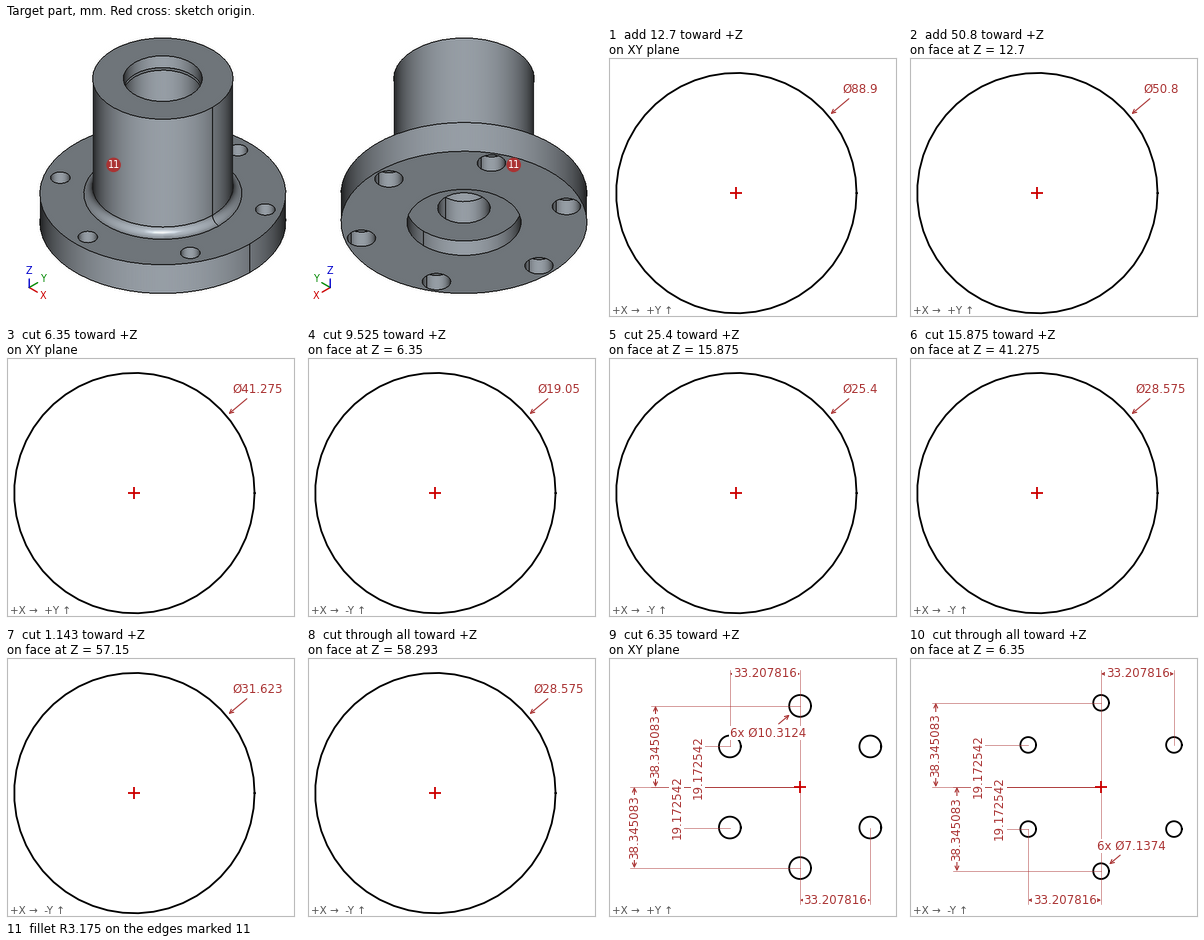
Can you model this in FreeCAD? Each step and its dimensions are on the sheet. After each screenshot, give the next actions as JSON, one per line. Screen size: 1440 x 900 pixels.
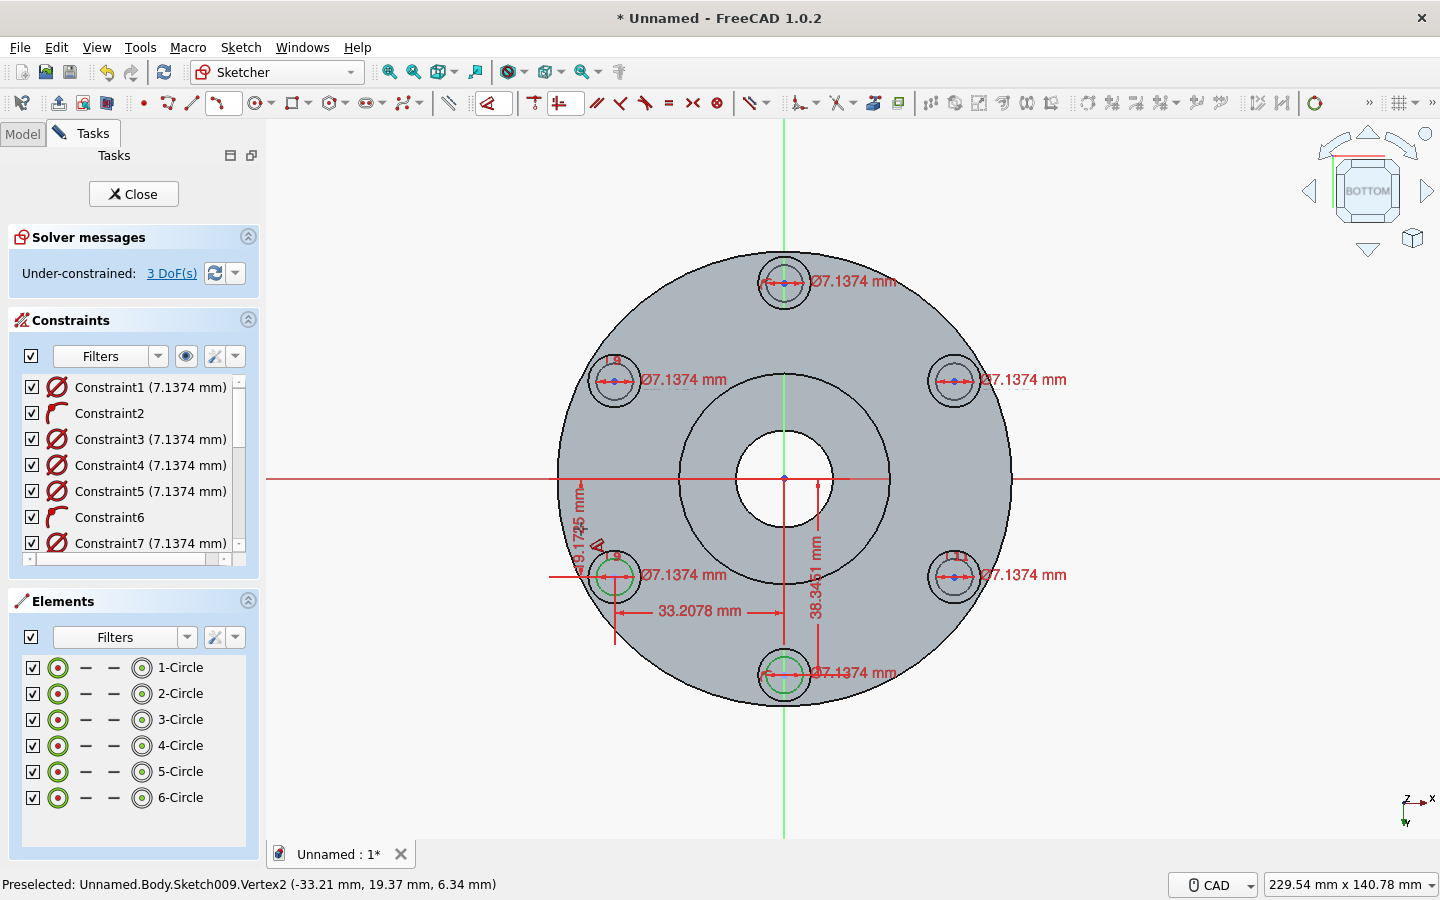
{"action": "left_click", "coordinate": [615, 382]}
{"action": "left_click", "coordinate": [581, 430]}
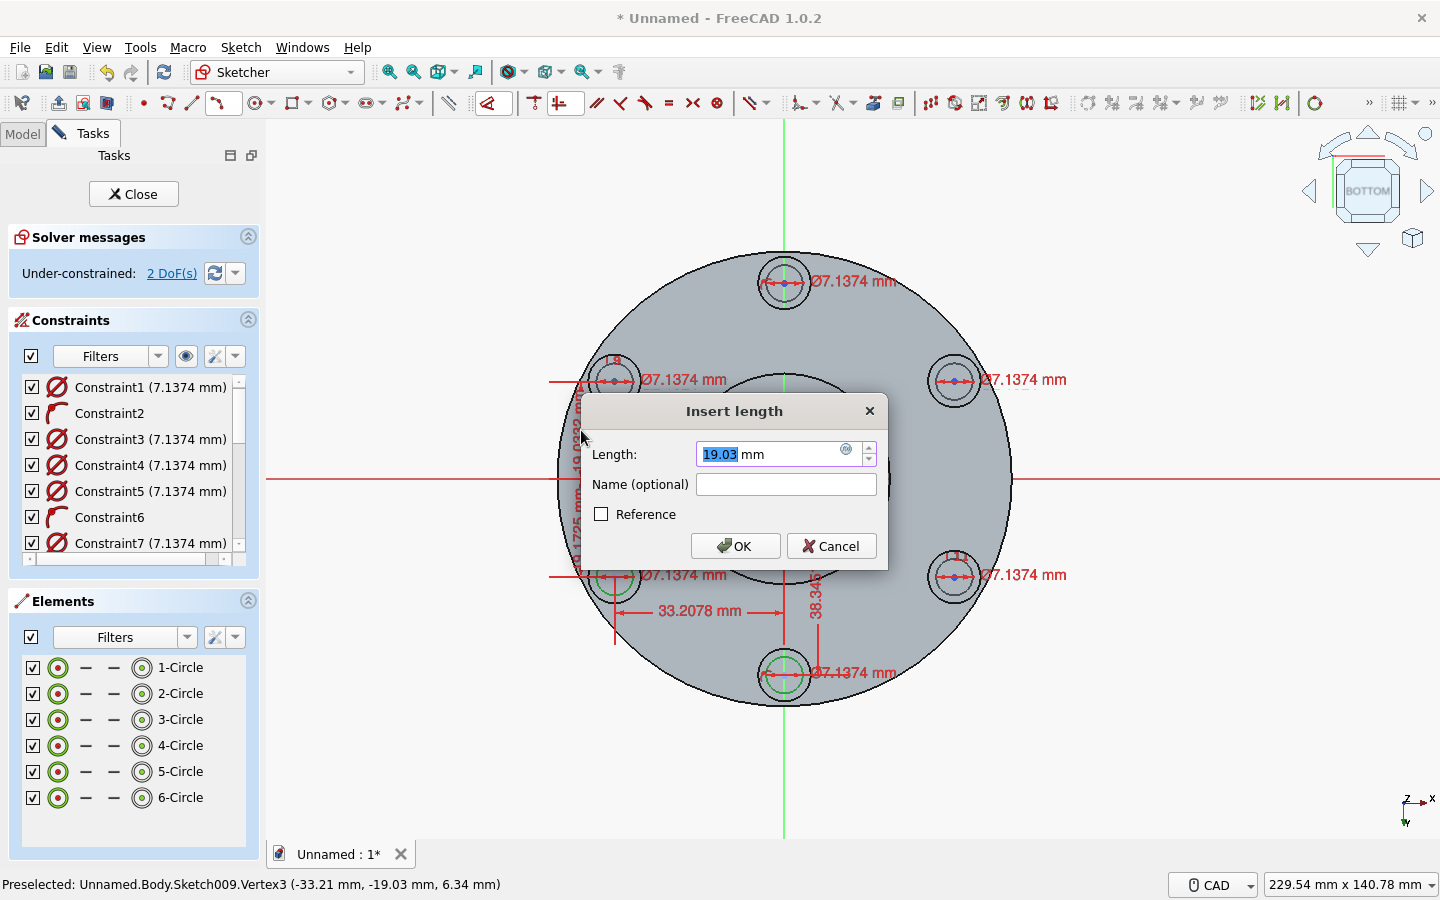
{"action": "type", "text": "19.172542"}
{"action": "key", "text": "Return"}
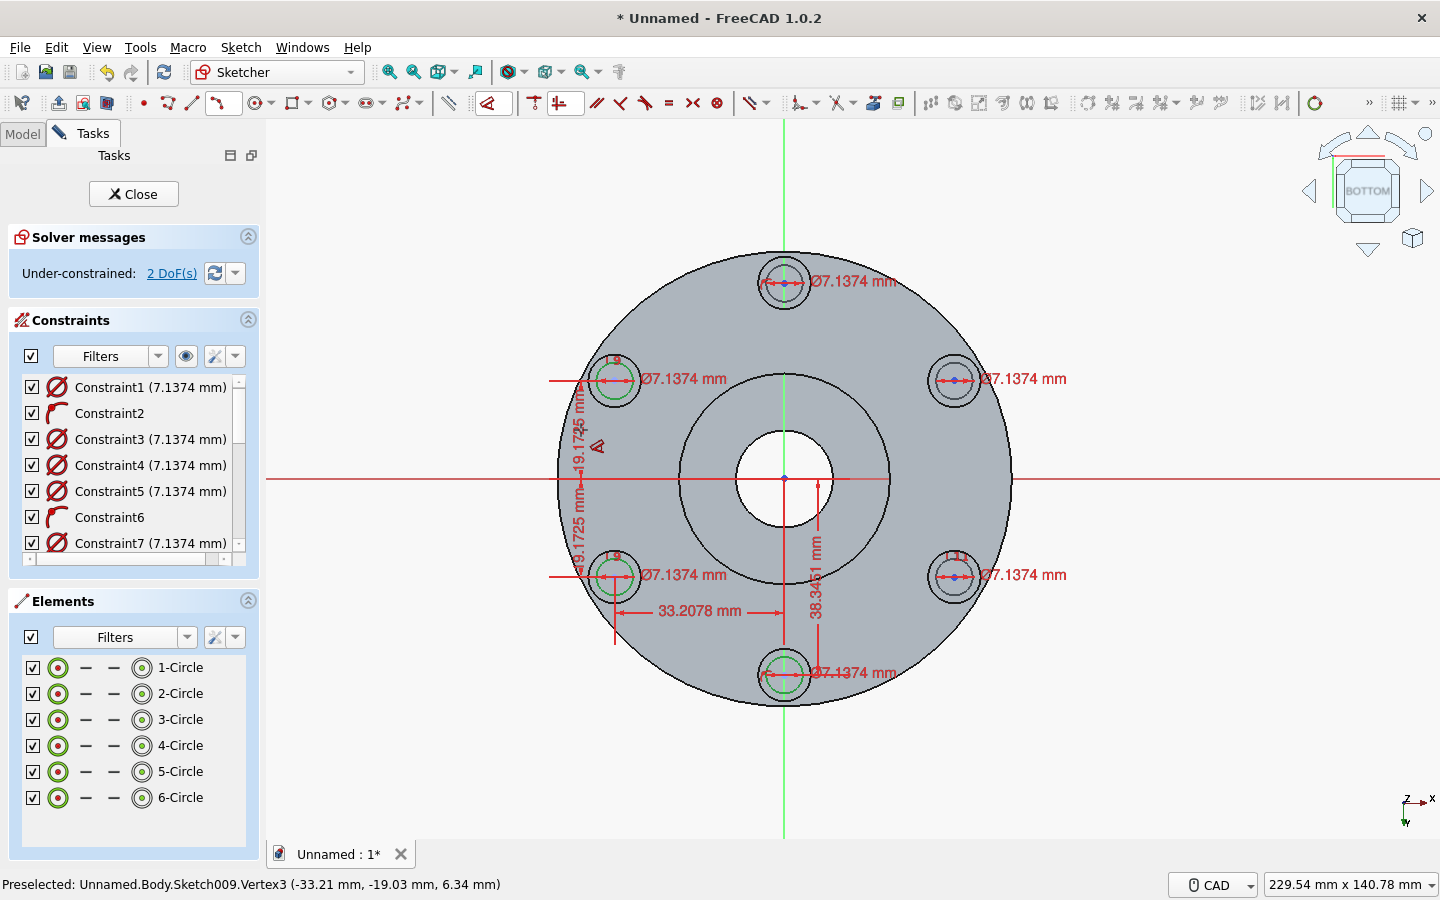
{"action": "left_click", "coordinate": [784, 283]}
{"action": "left_click", "coordinate": [818, 381]}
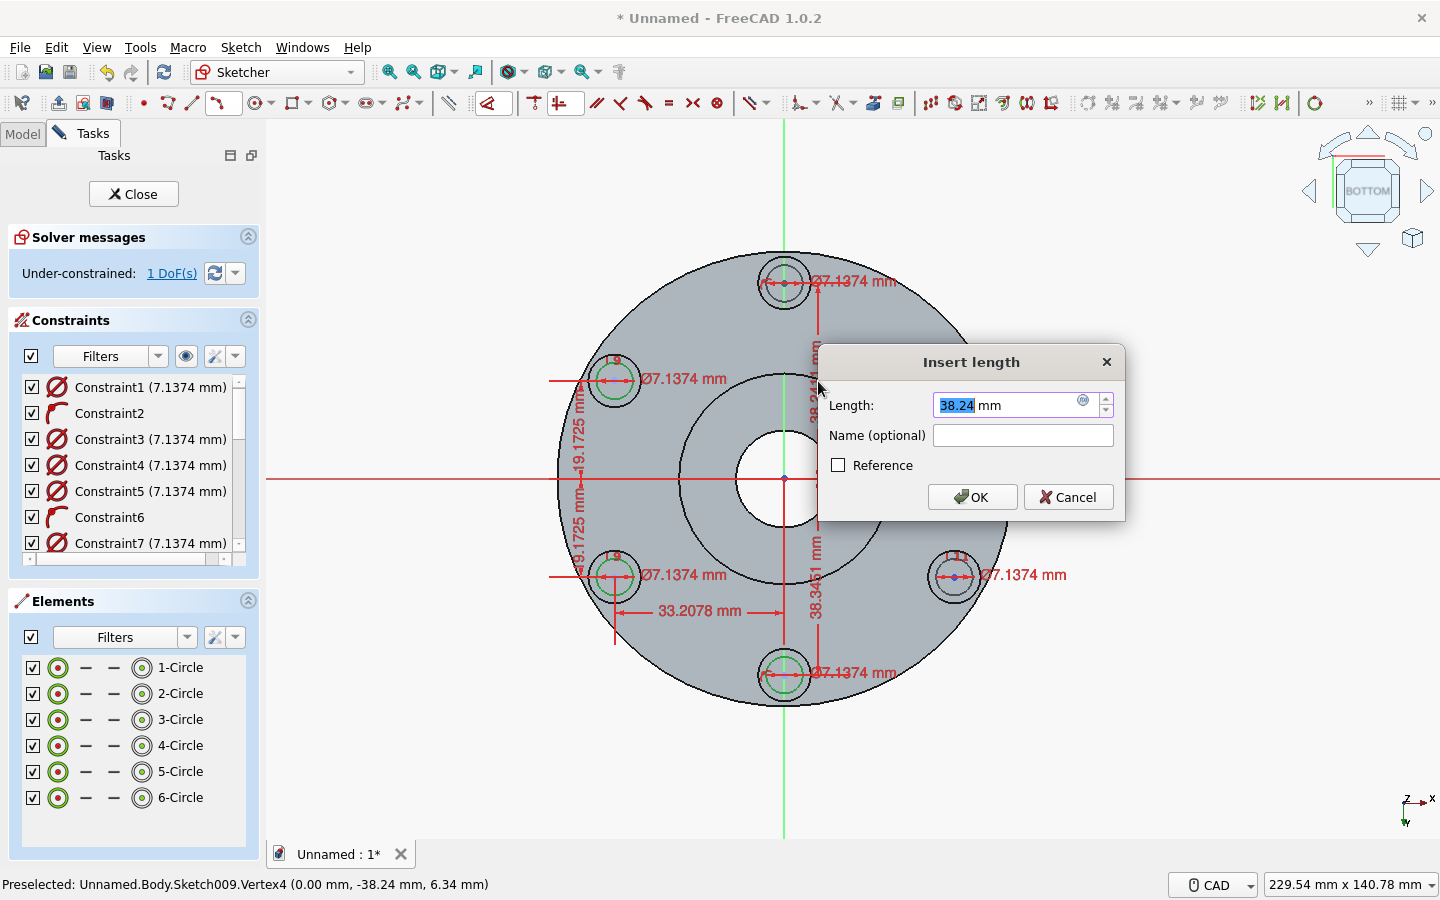
{"action": "type", "text": "38.345083"}
{"action": "key", "text": "Return"}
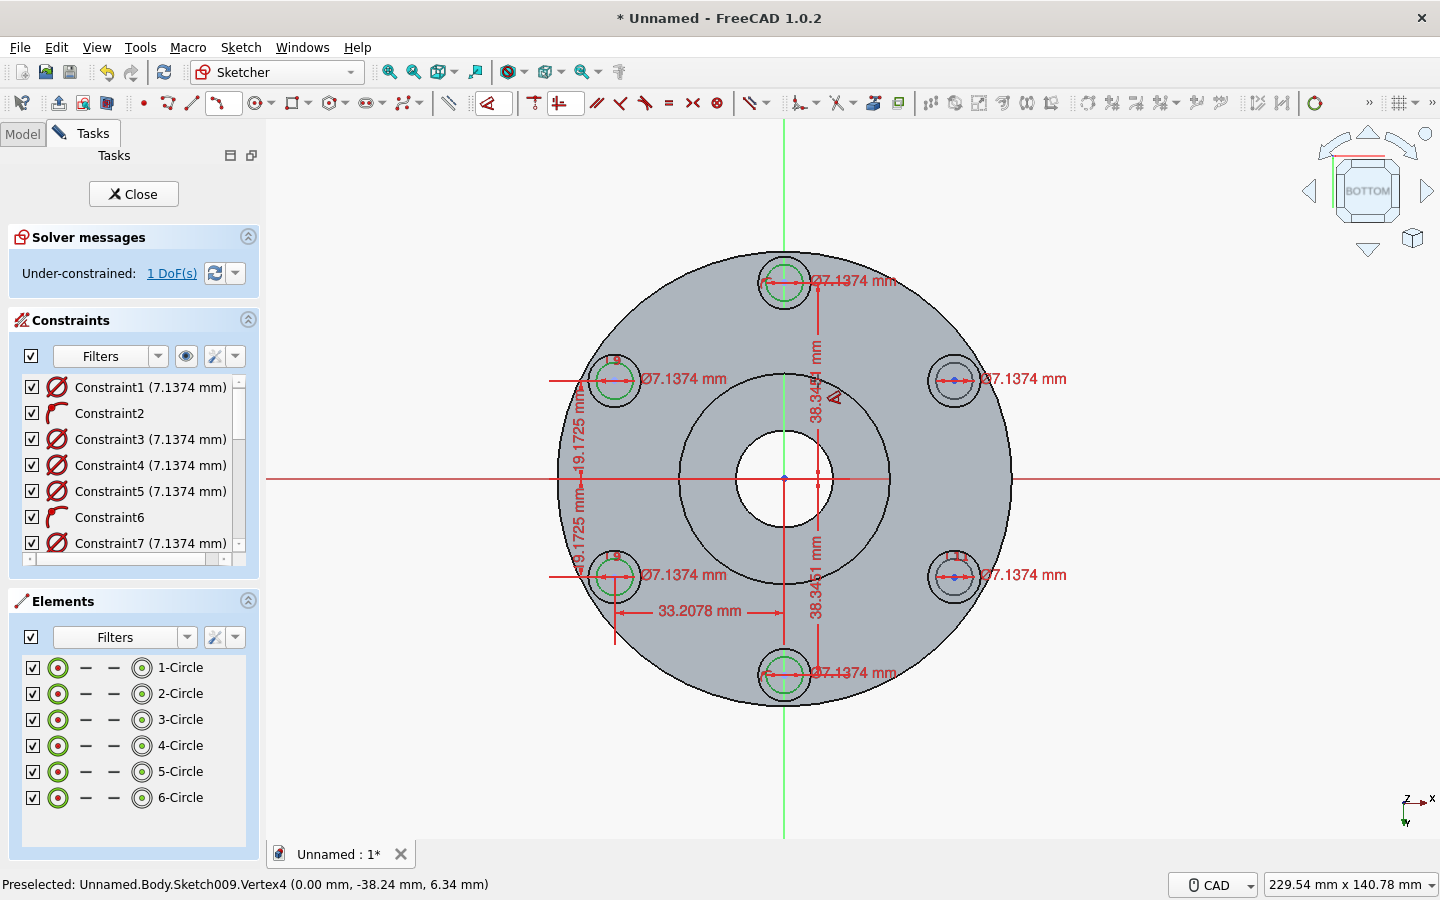
{"action": "left_click", "coordinate": [954, 381]}
{"action": "left_click", "coordinate": [869, 347]}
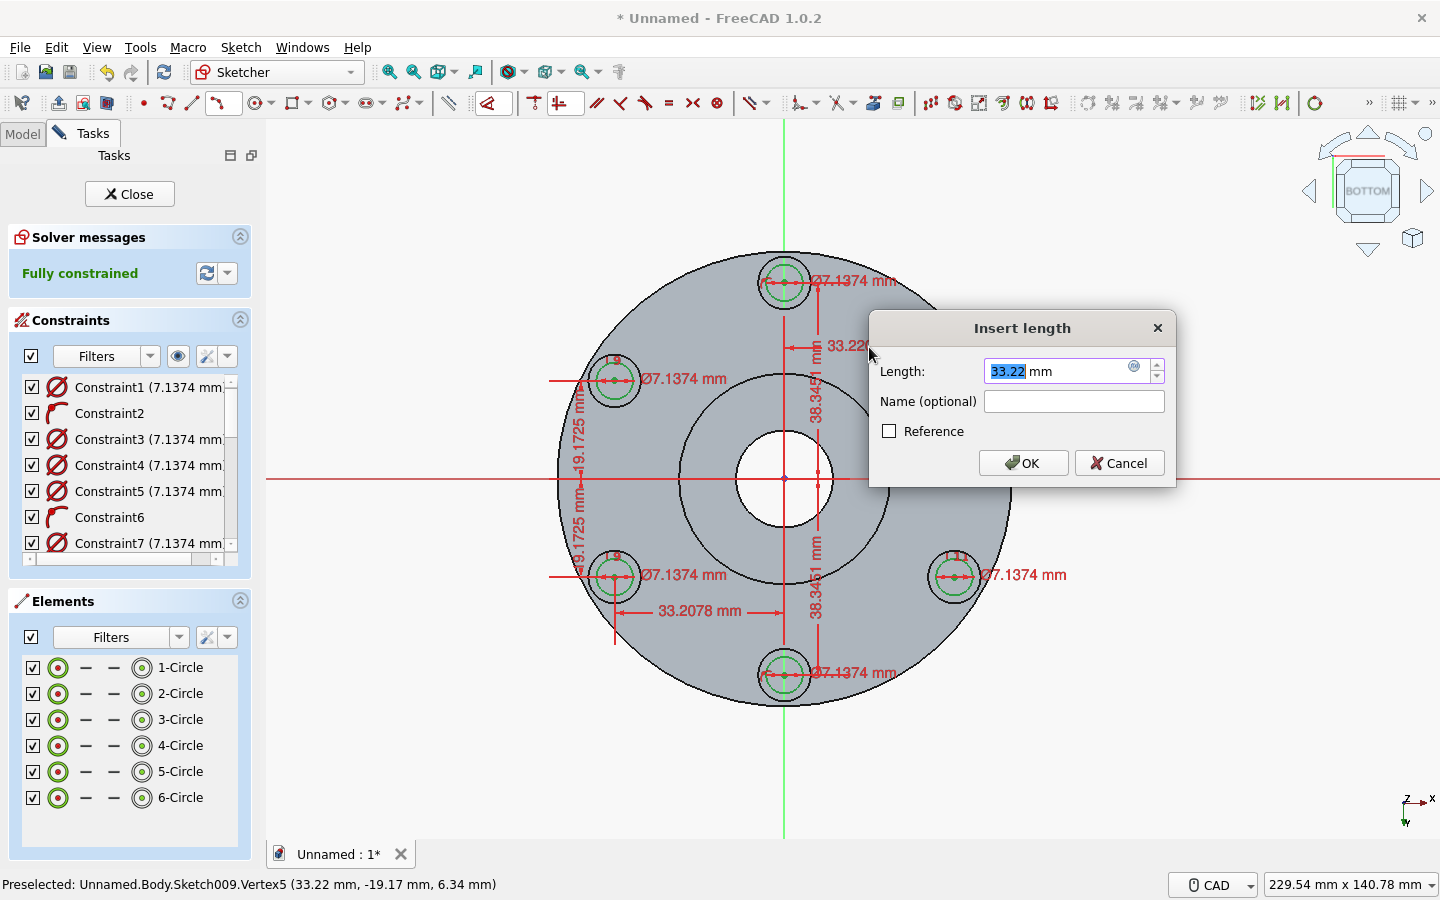
{"action": "type", "text": "33.207816"}
{"action": "key", "text": "Return"}
{"action": "key", "text": "Escape"}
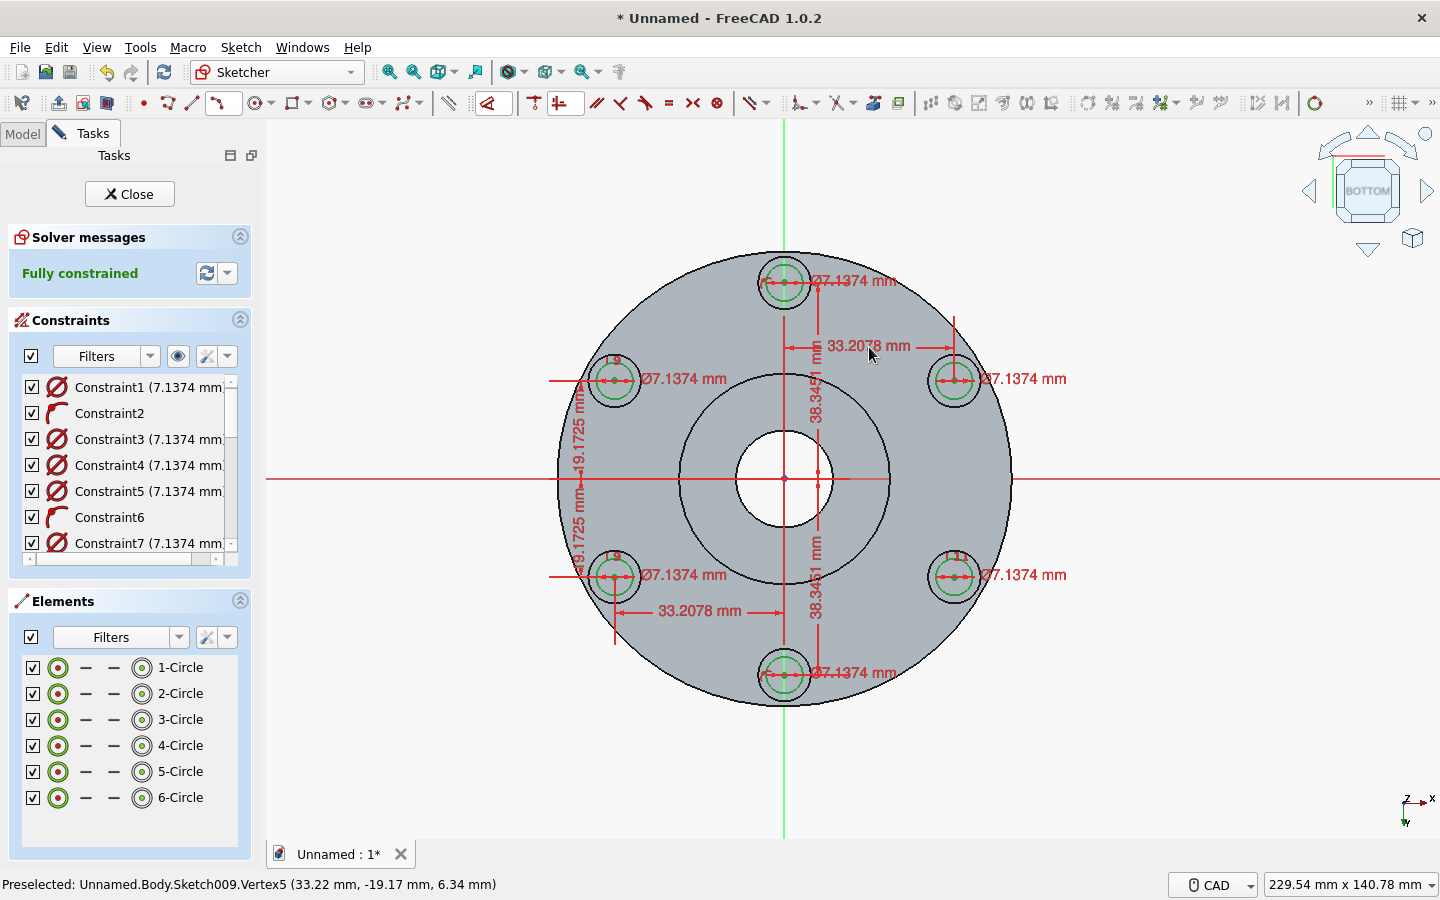
{"action": "left_click", "coordinate": [130, 194]}